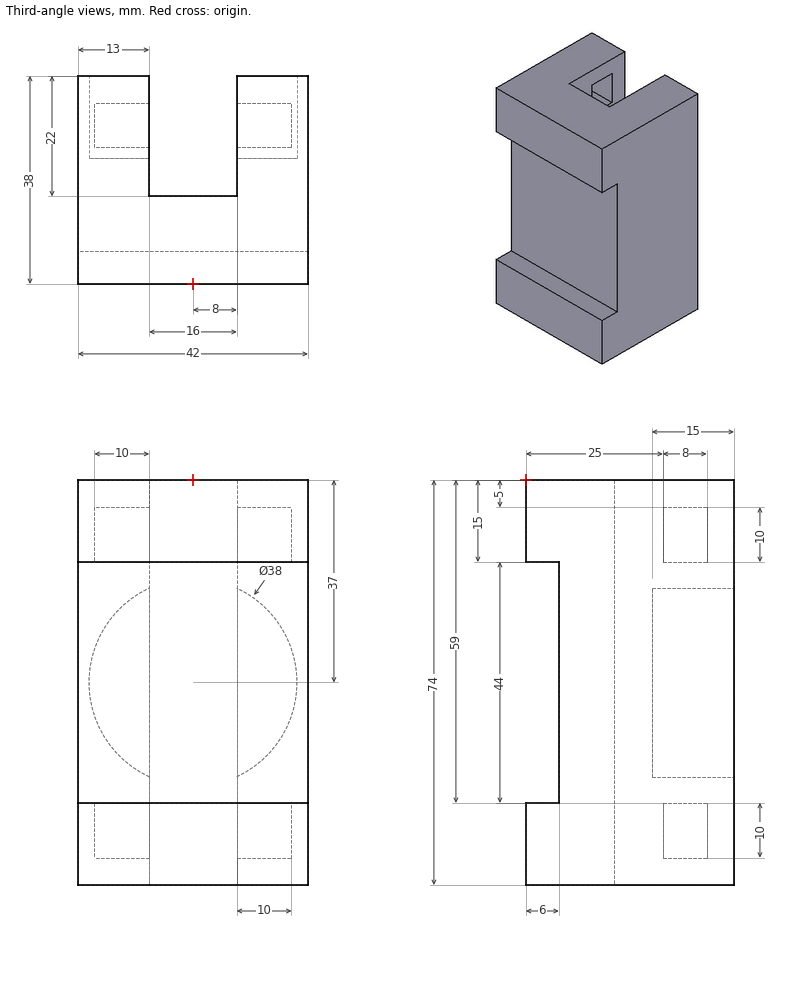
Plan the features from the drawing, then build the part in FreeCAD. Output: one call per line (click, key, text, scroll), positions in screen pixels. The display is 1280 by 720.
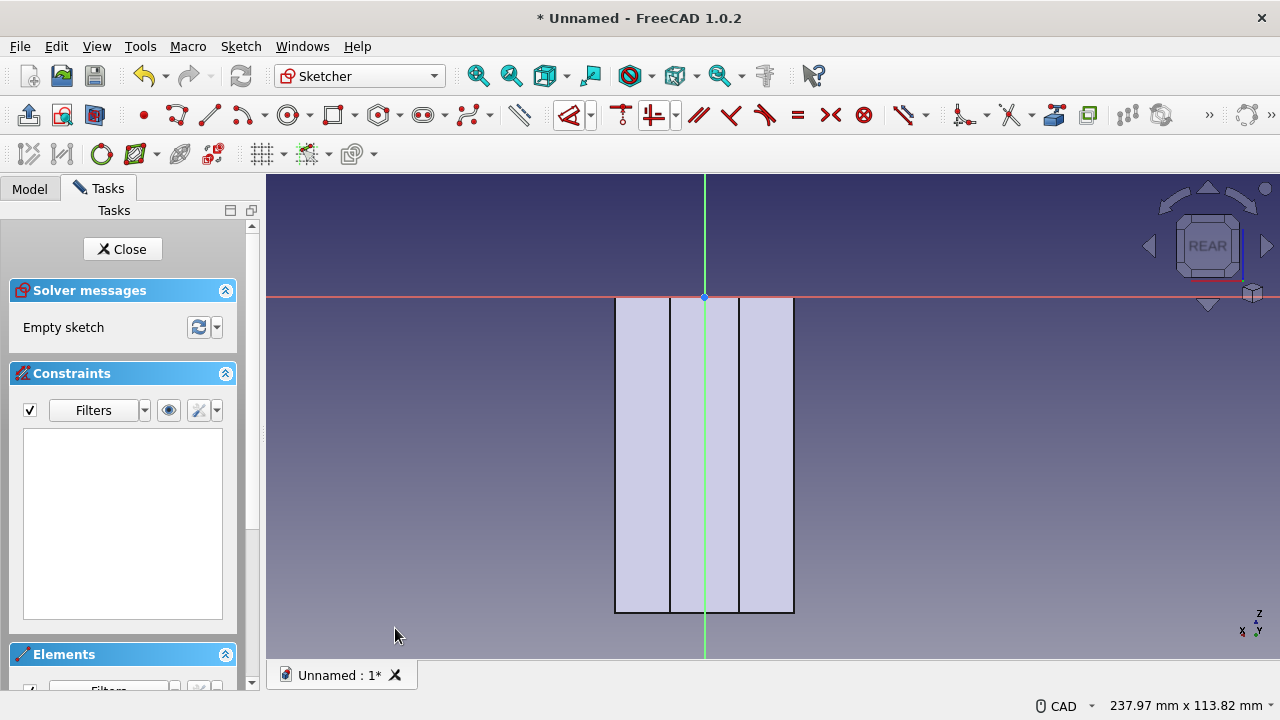
key(g)
key(c)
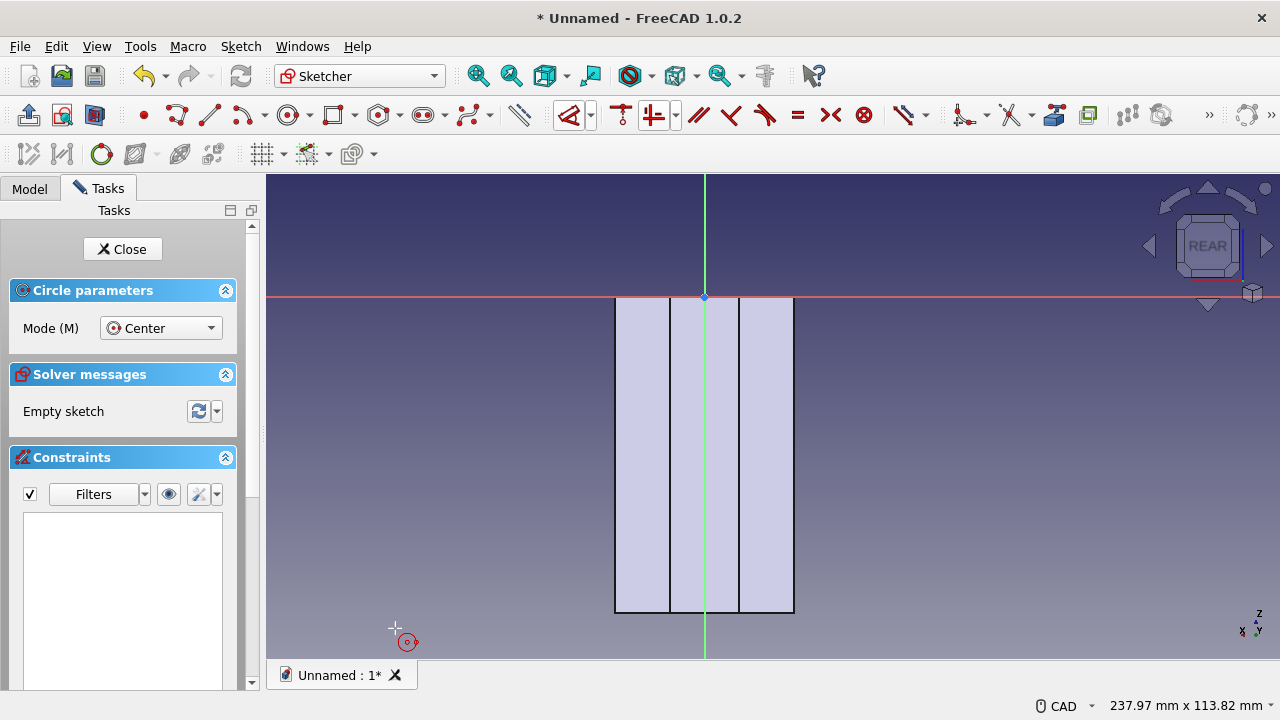
click(705, 455)
move(762, 398)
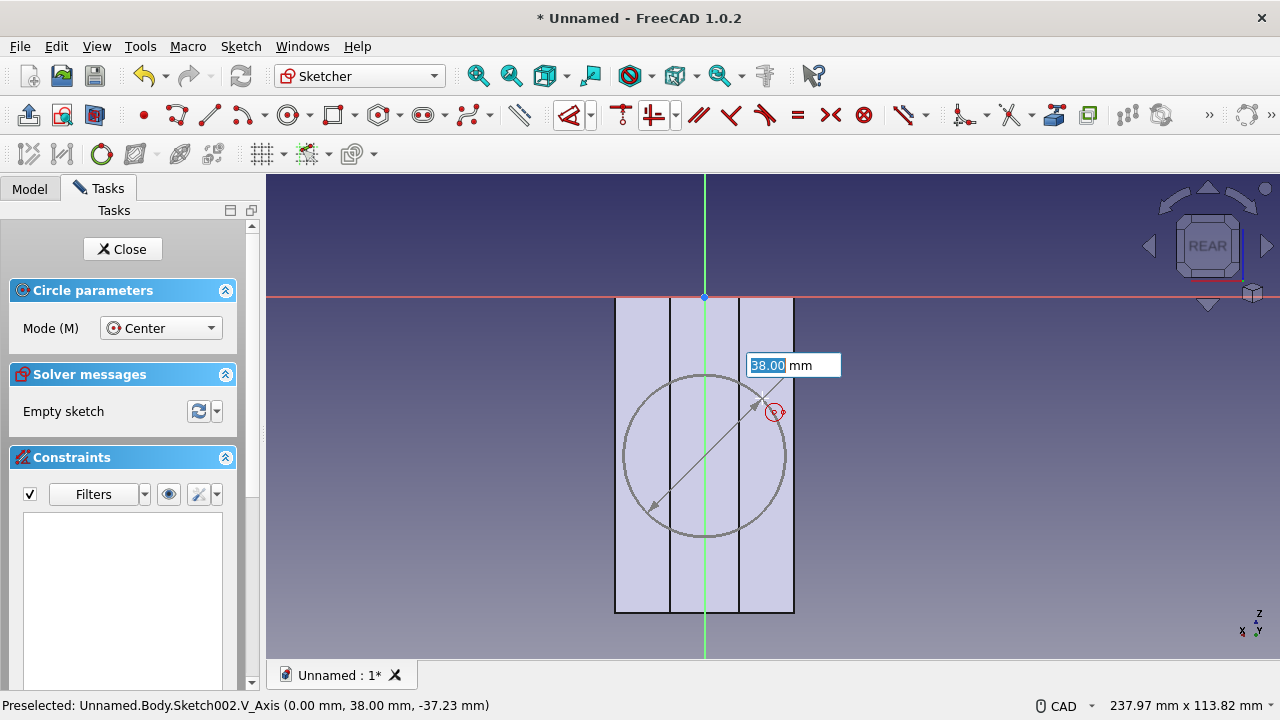
text(38)
key(Return)
key(Escape)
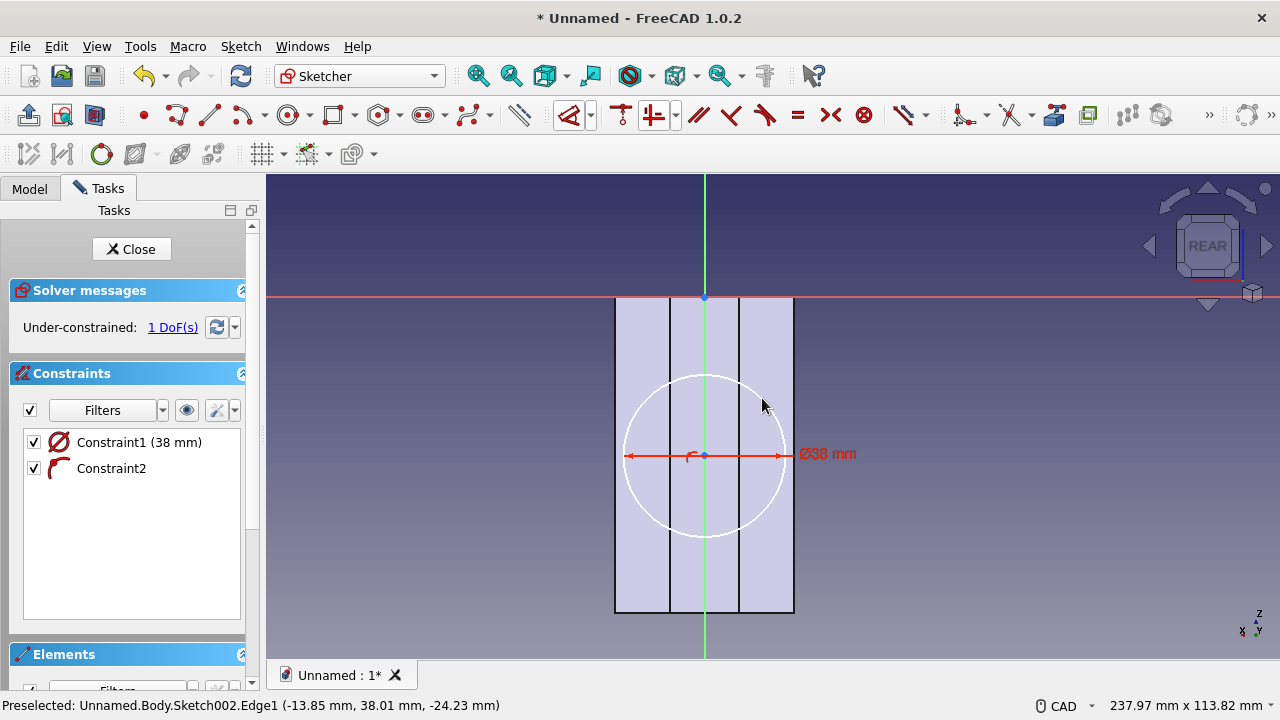
click(705, 456)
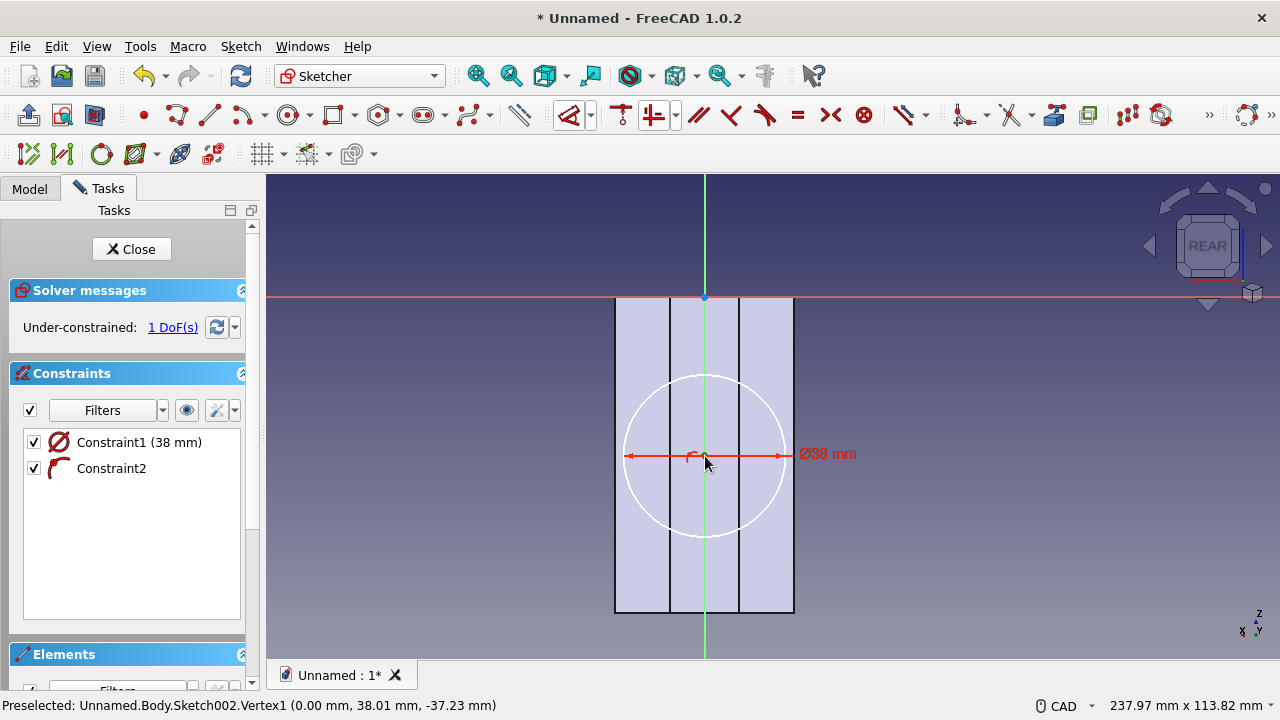
key(i)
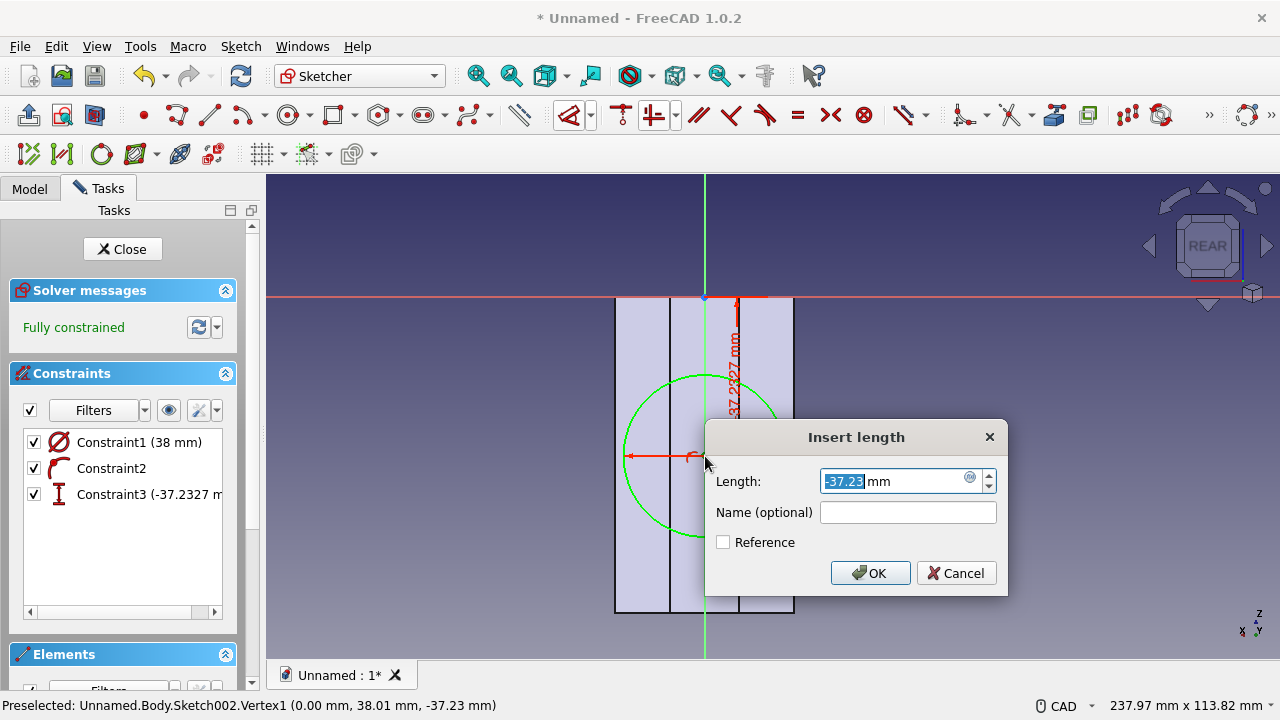
text(-37)
key(Return)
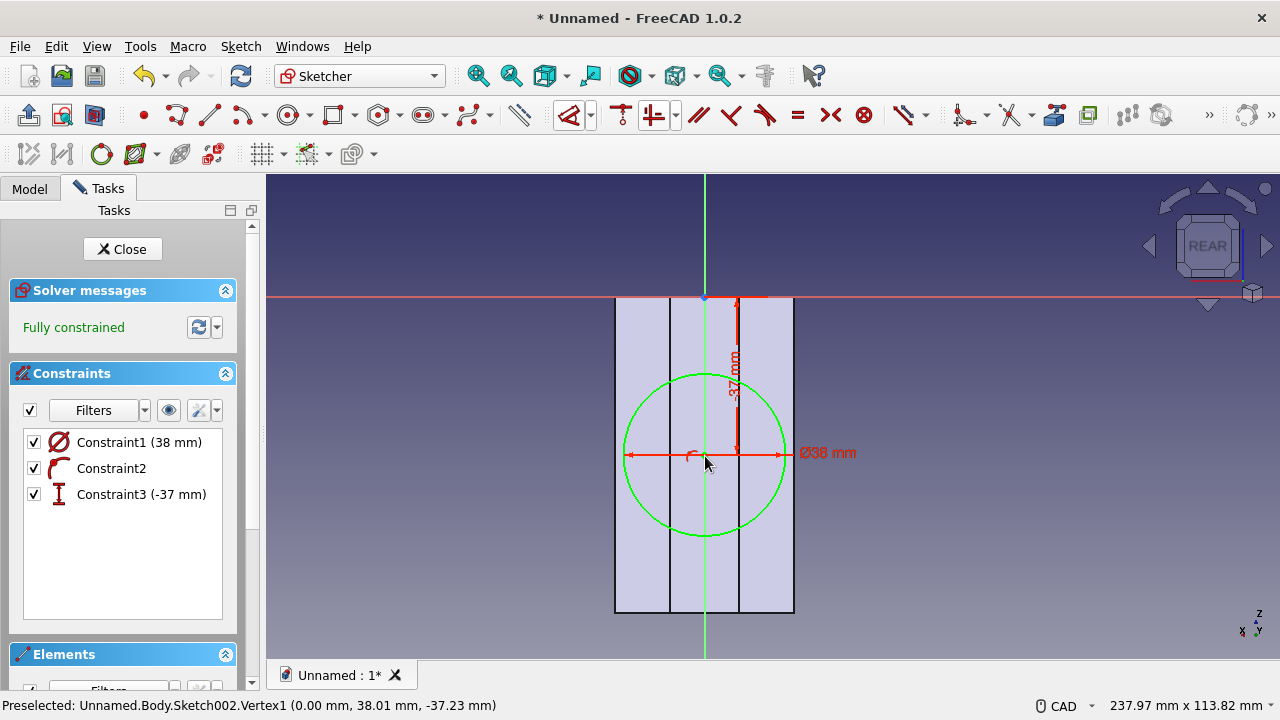
click(123, 249)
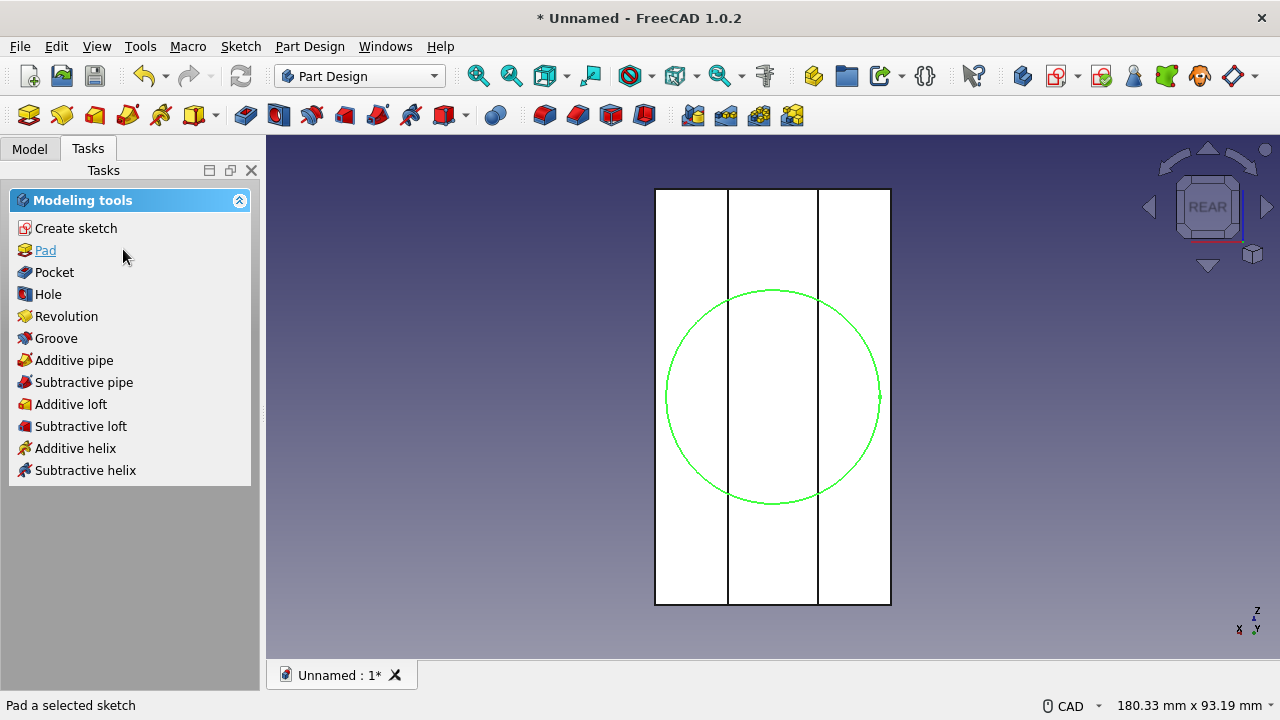
click(246, 116)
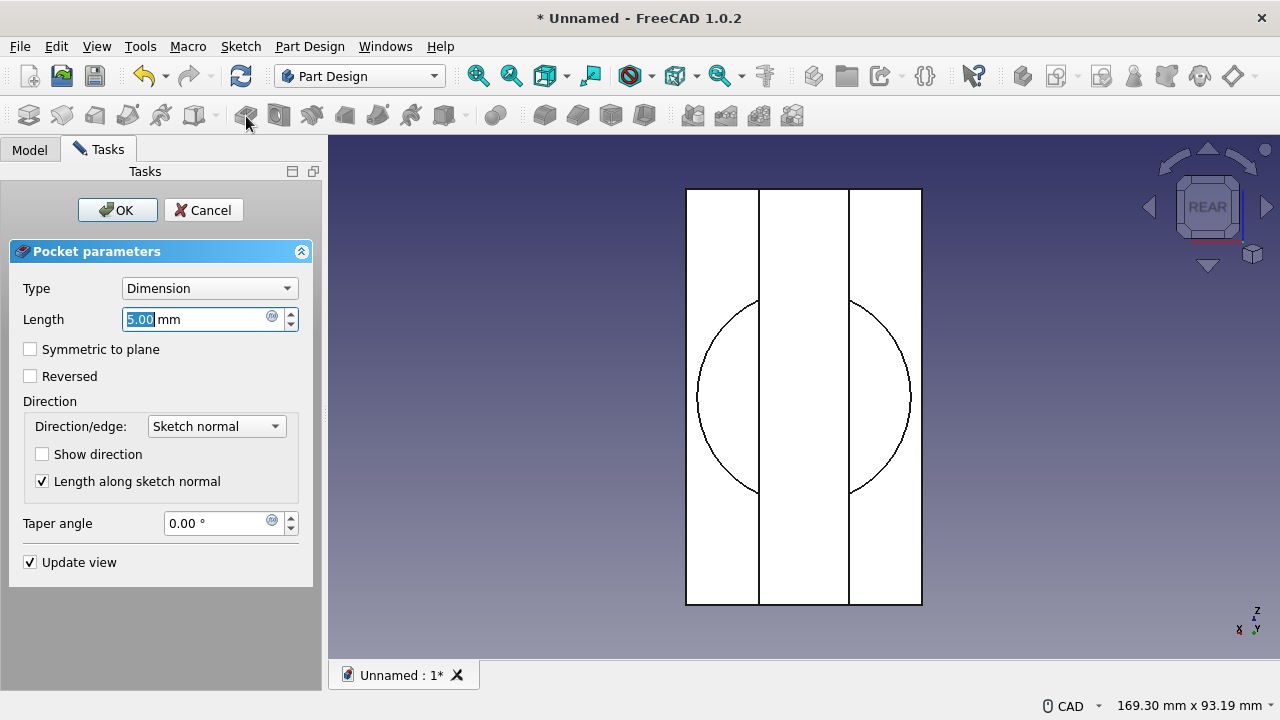
text(15)
key(Tab)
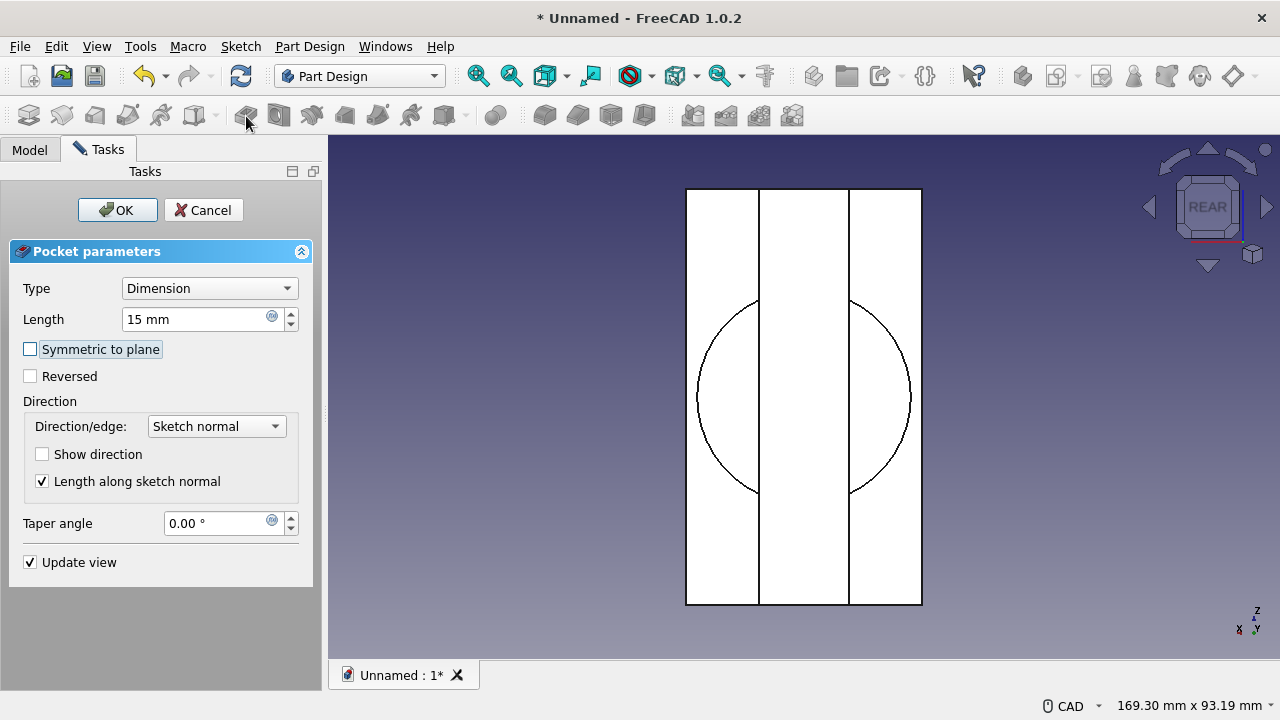
click(118, 210)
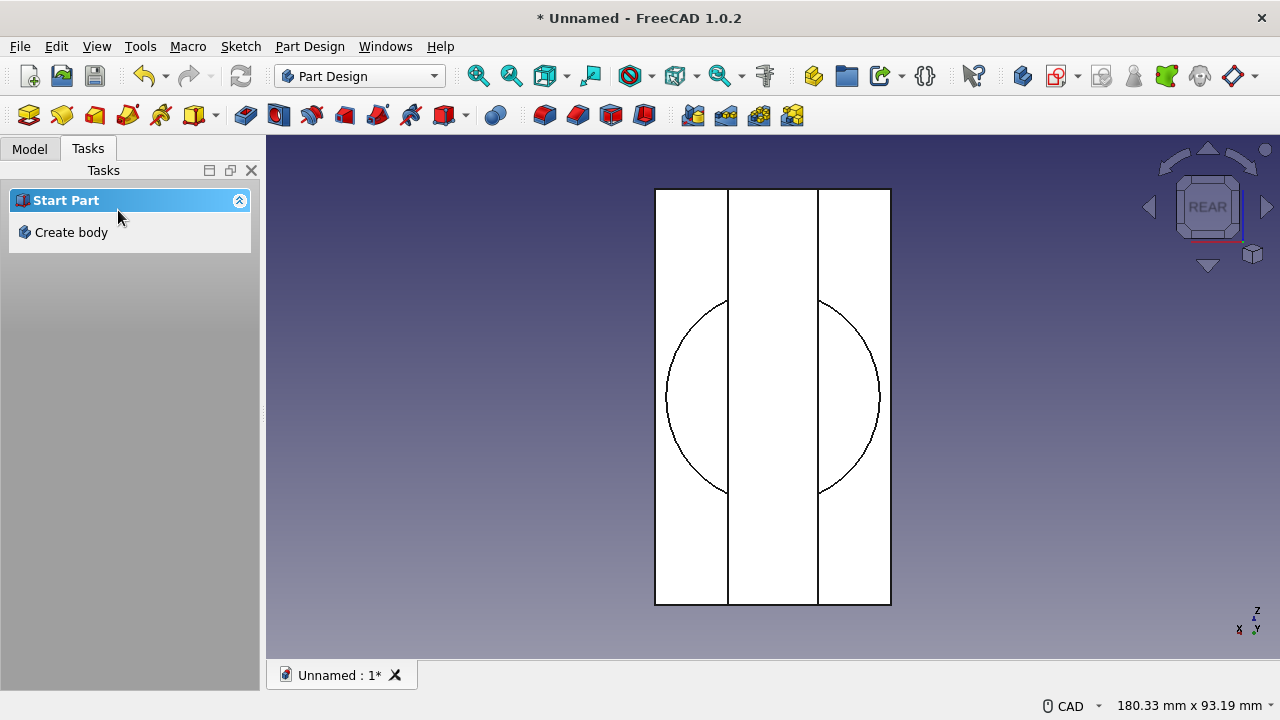
click(30, 148)